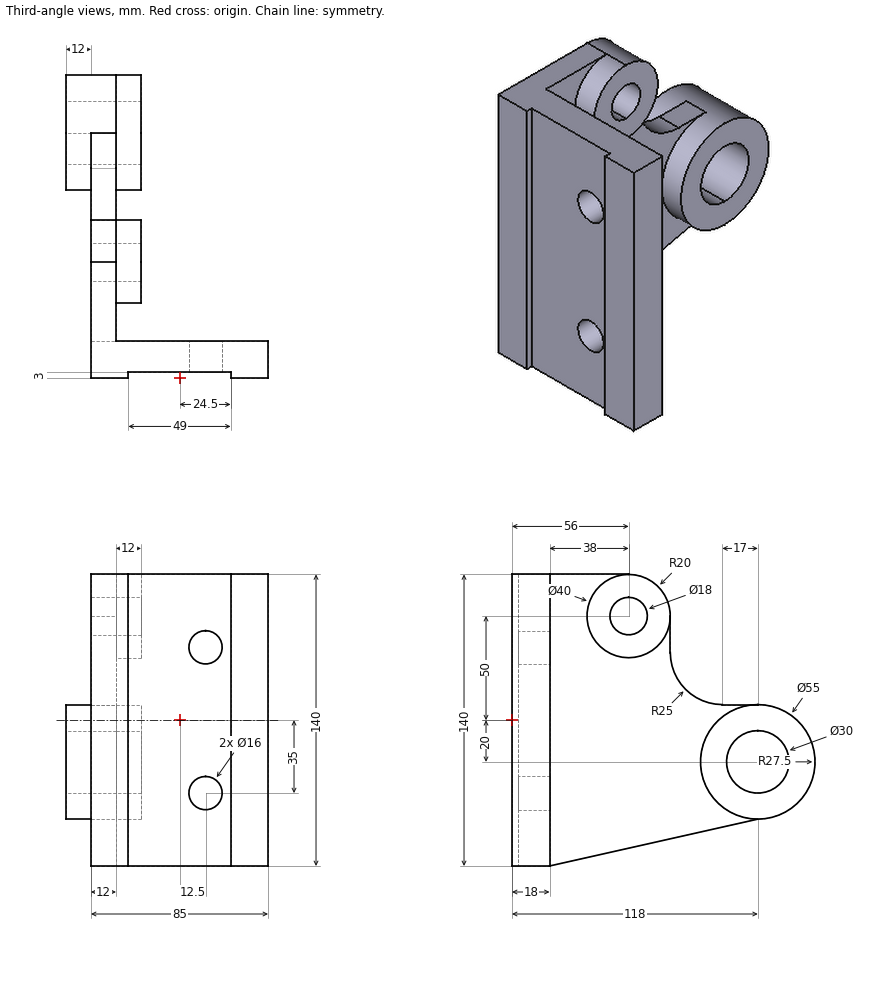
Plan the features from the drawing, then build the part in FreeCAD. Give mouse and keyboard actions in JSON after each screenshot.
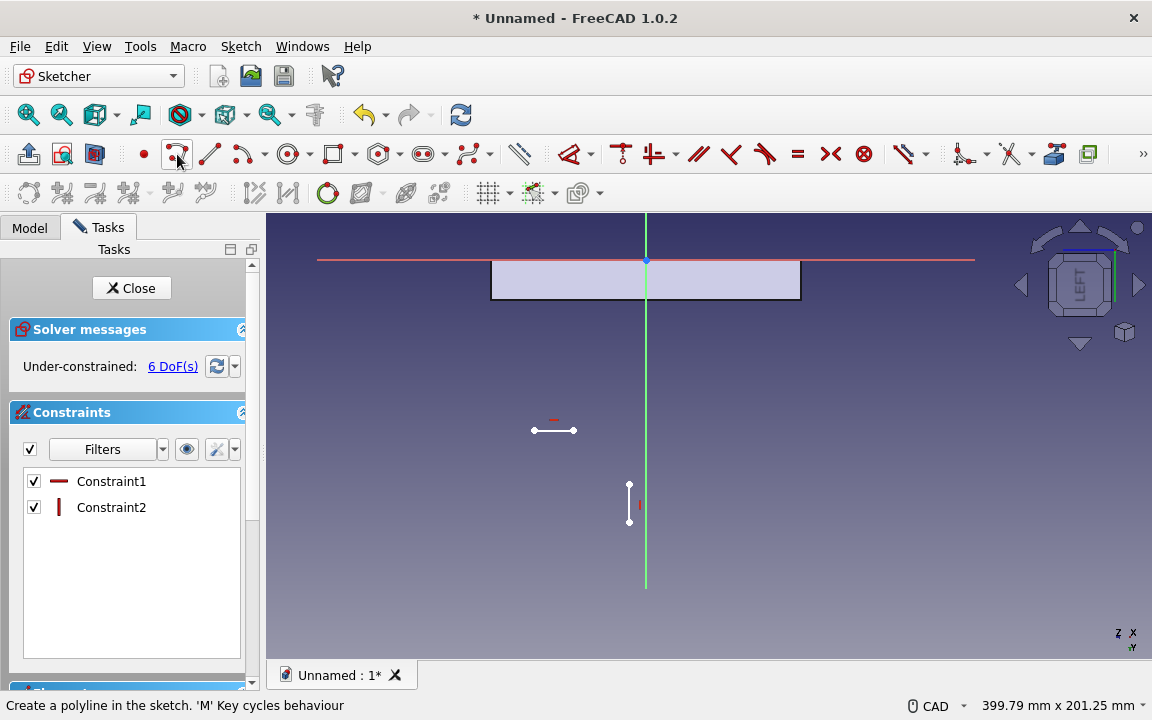
{"action": "left_click", "coordinate": [751, 522]}
{"action": "left_click", "coordinate": [801, 300]}
{"action": "left_click", "coordinate": [491, 300]}
{"action": "left_click", "coordinate": [491, 385]}
{"action": "right_click", "coordinate": [491, 385]}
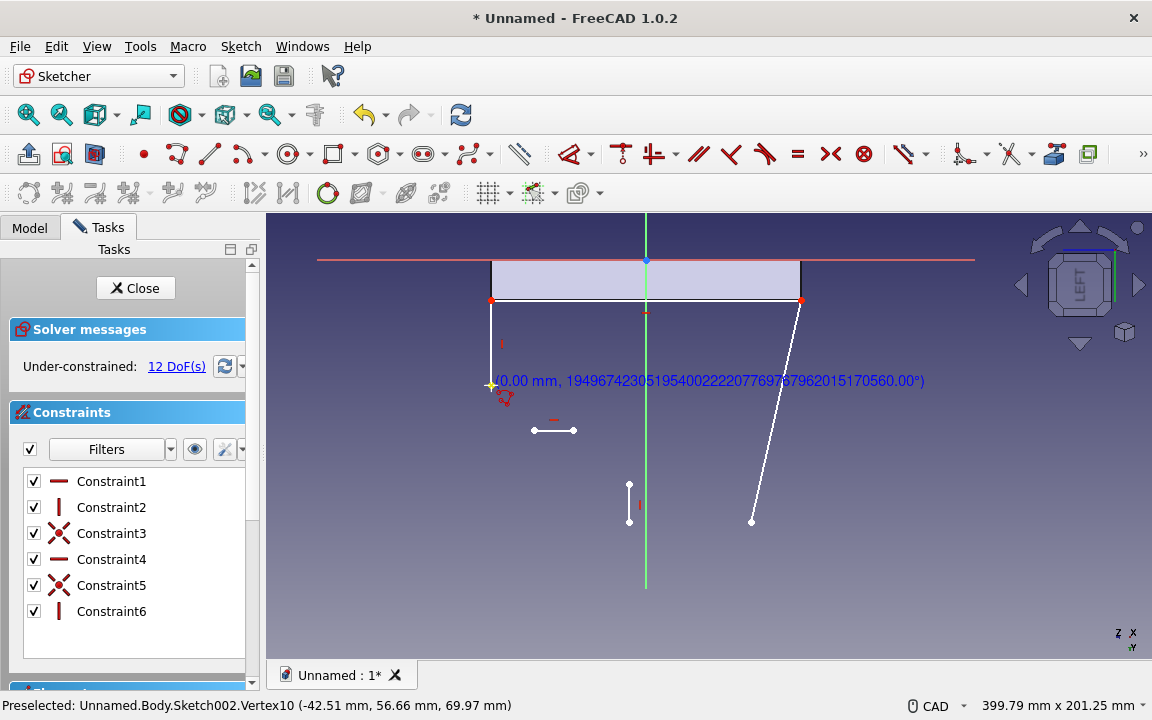
{"action": "key", "text": "g 3 a"}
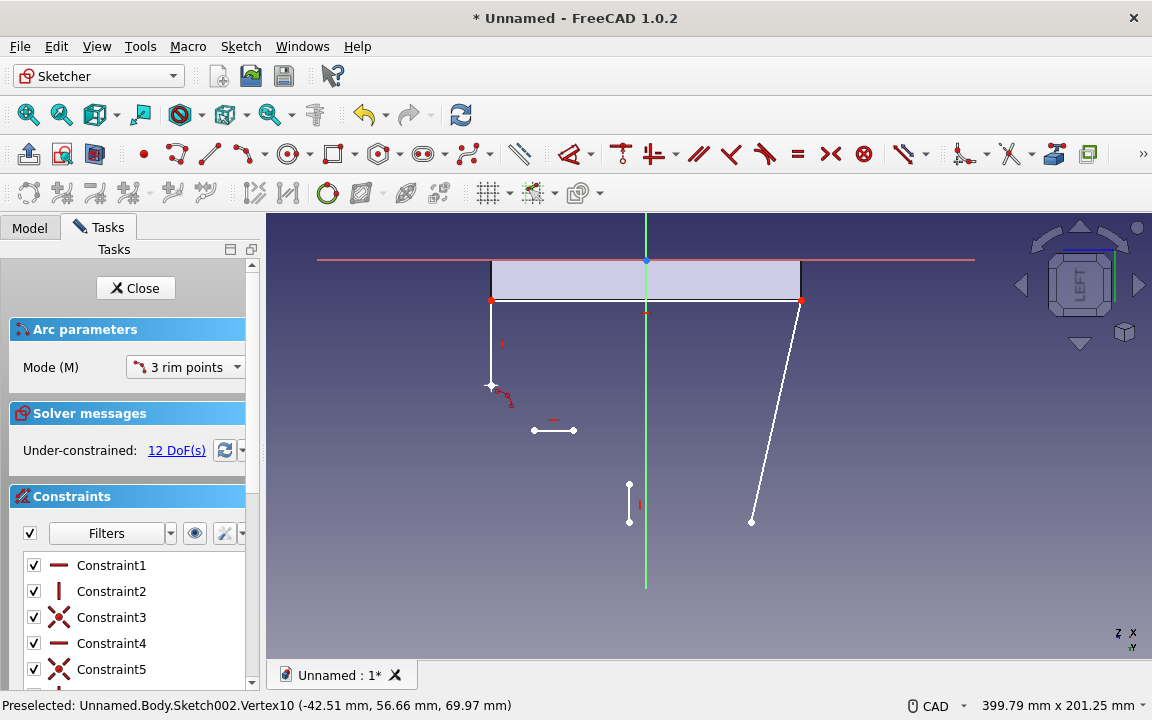
{"action": "left_click", "coordinate": [574, 431]}
{"action": "left_click", "coordinate": [629, 485]}
{"action": "left_click", "coordinate": [613, 445]}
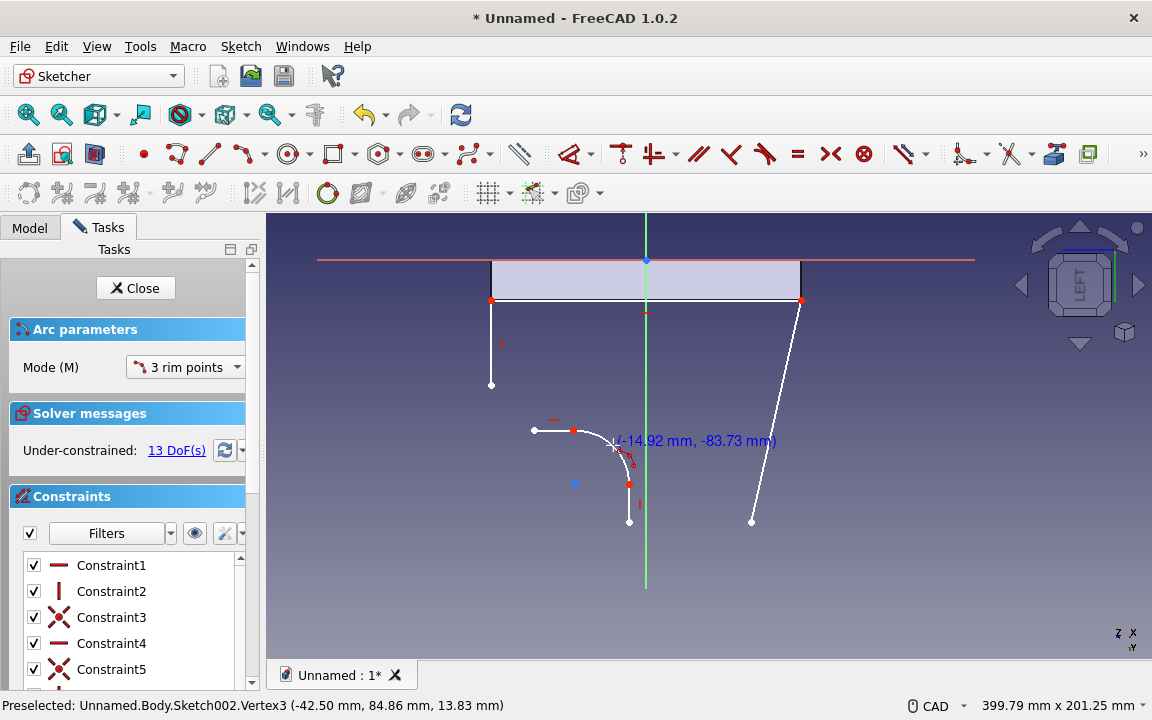
{"action": "left_click", "coordinate": [629, 523]}
{"action": "left_click", "coordinate": [751, 523]}
{"action": "left_click", "coordinate": [690, 583]}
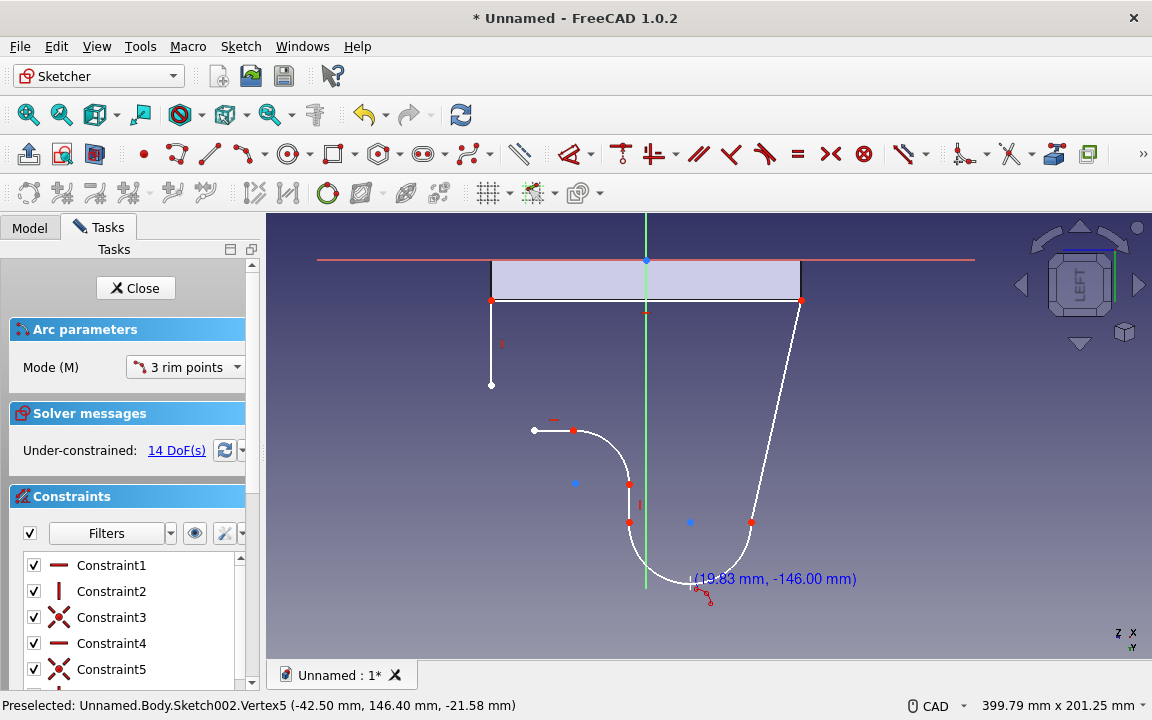
{"action": "left_click", "coordinate": [491, 386]}
{"action": "left_click", "coordinate": [535, 431]}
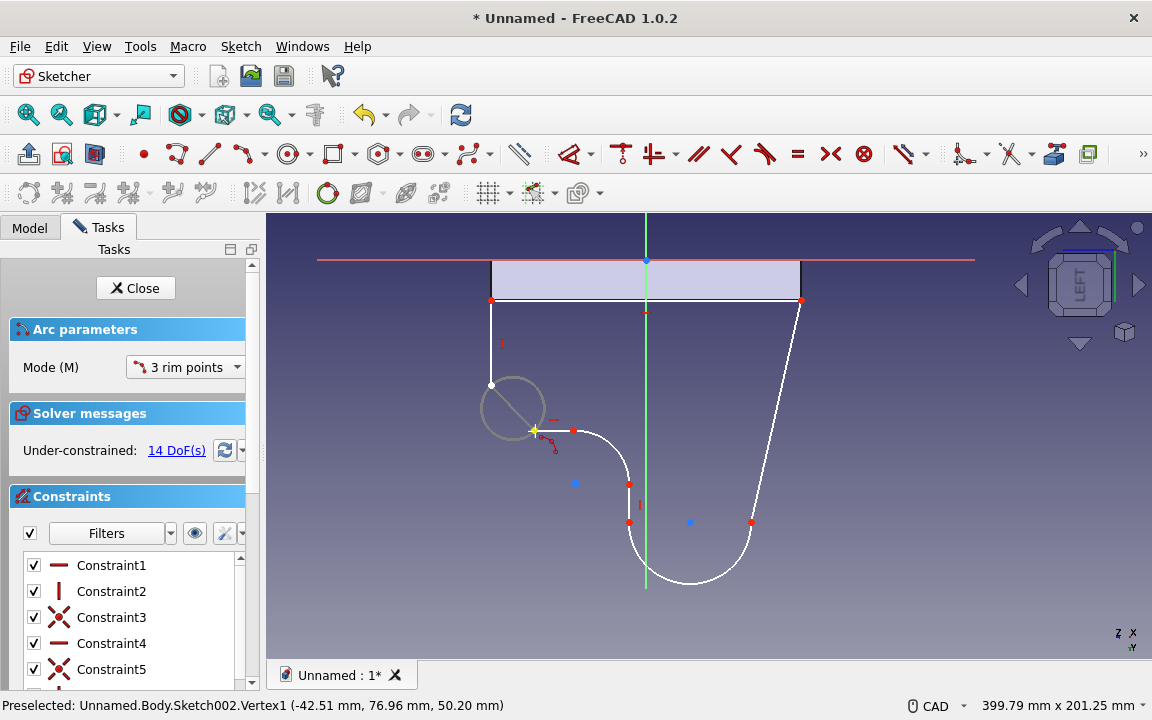
{"action": "scroll", "coordinate": [504, 416], "scroll_direction": "up", "scroll_amount": 2}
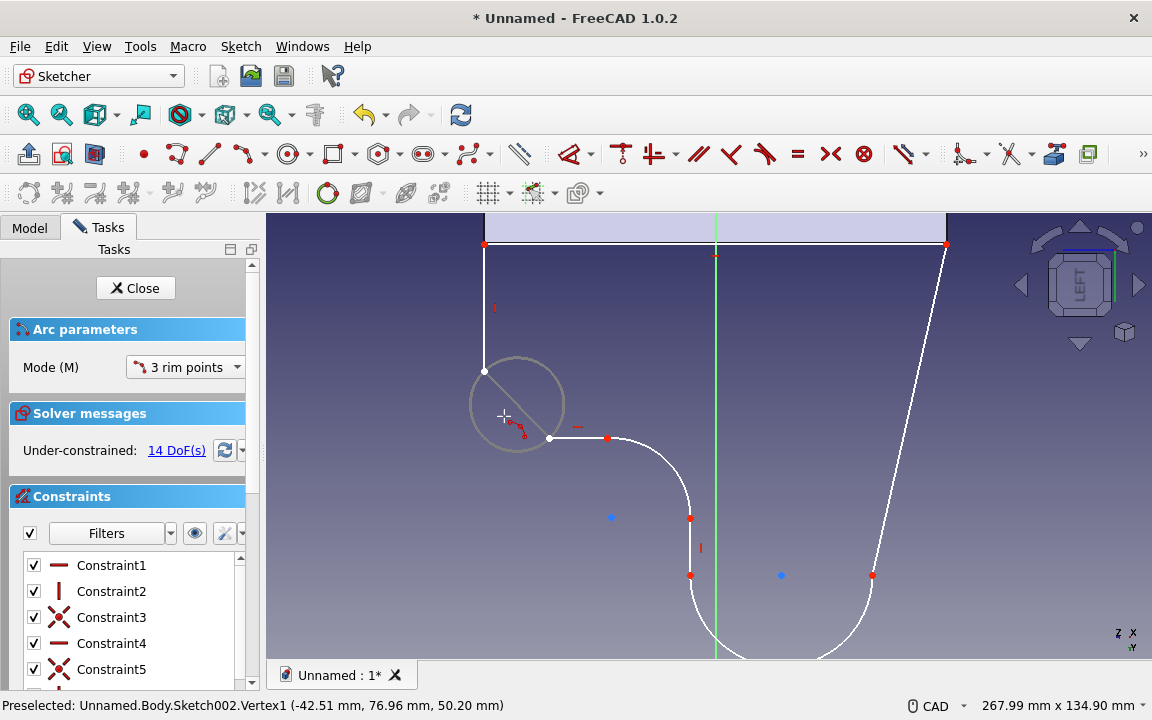
{"action": "left_click", "coordinate": [504, 416]}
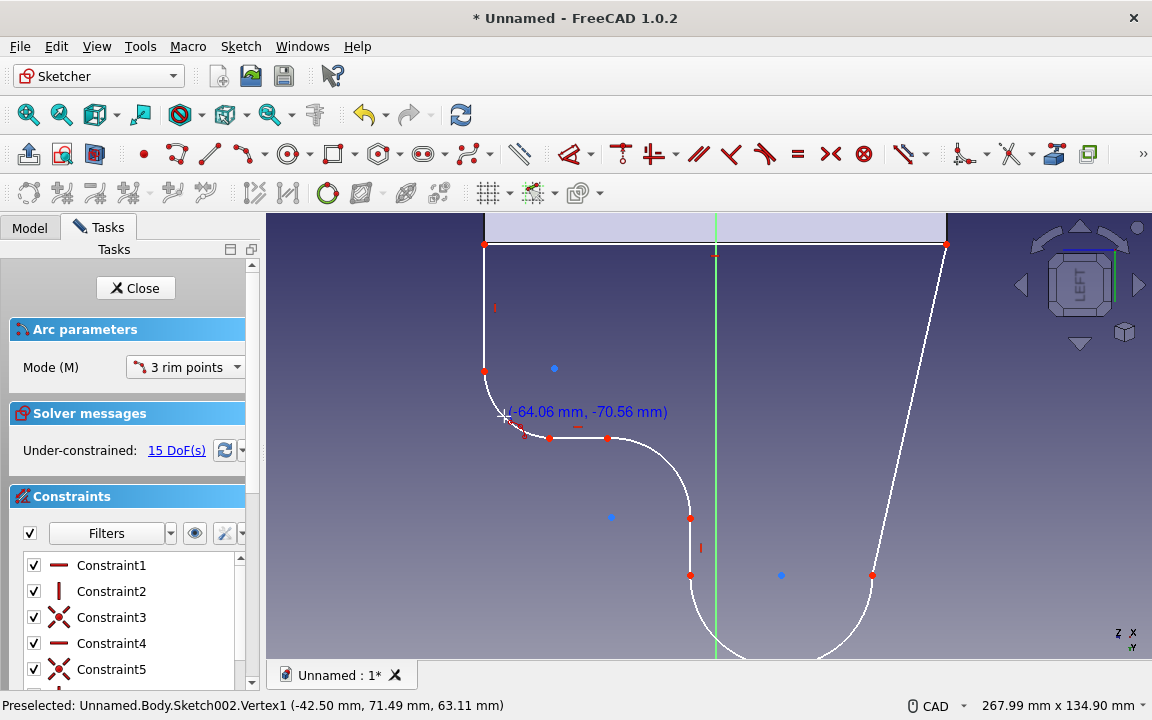
{"action": "key", "text": "g c"}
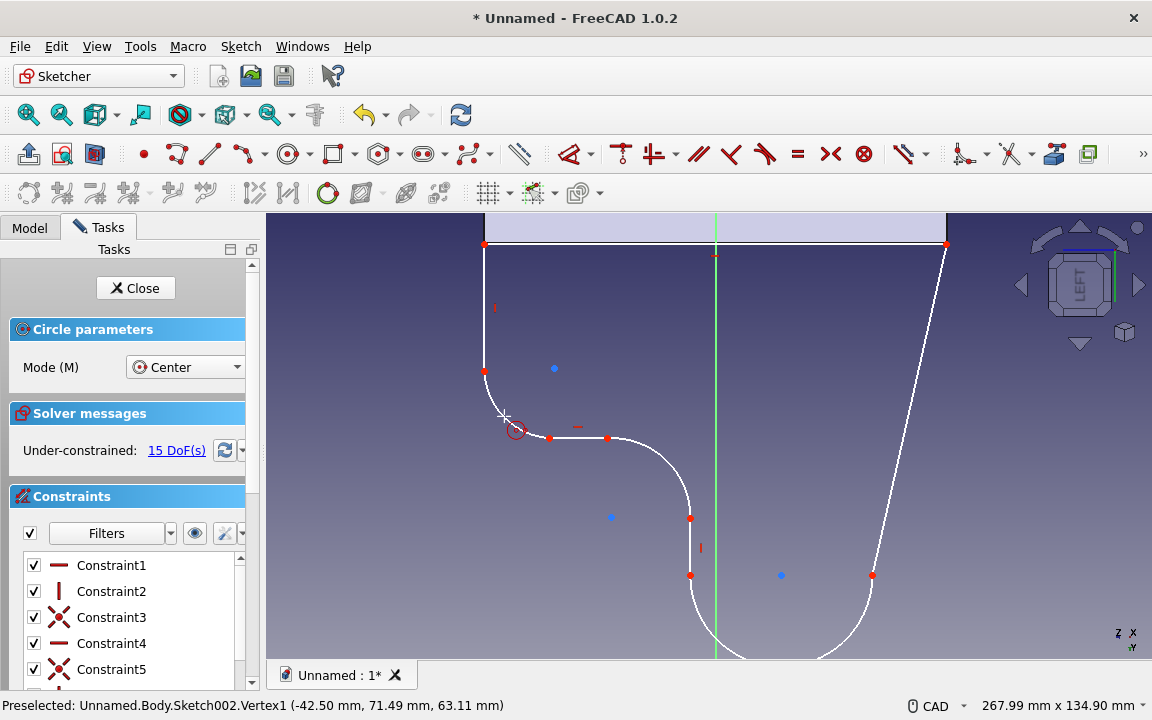
{"action": "left_click", "coordinate": [550, 369]}
{"action": "mouse_move", "coordinate": [572, 348]}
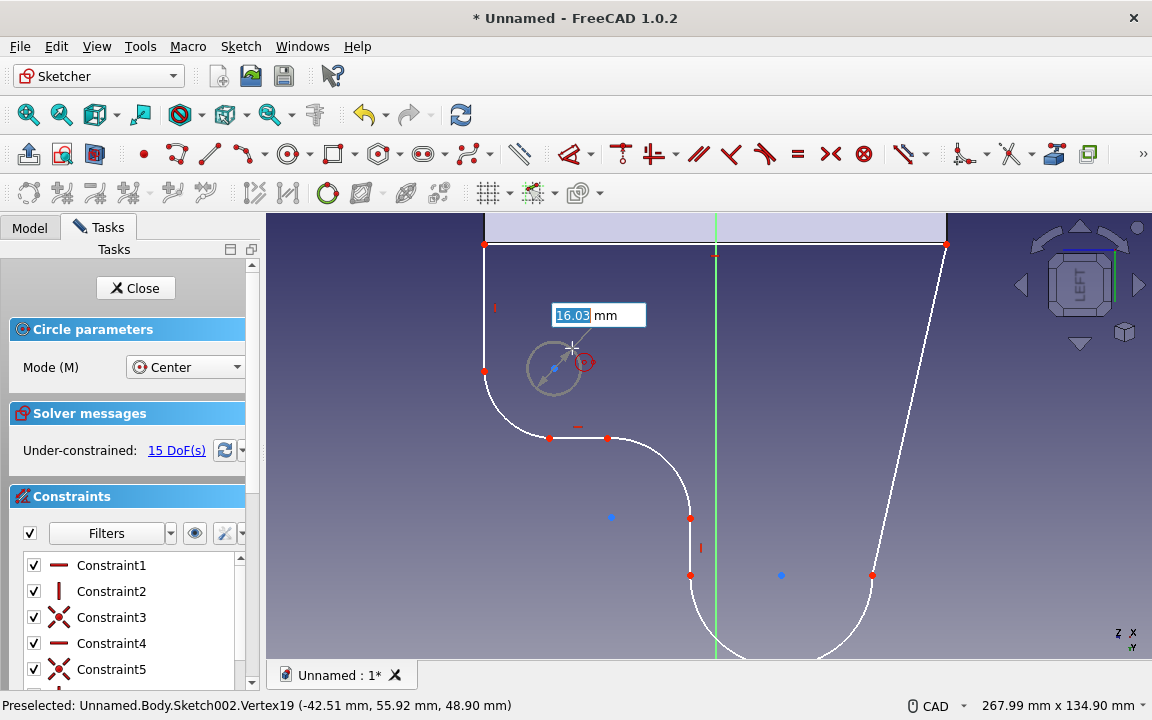
{"action": "type", "text": "18"}
{"action": "key", "text": "Return"}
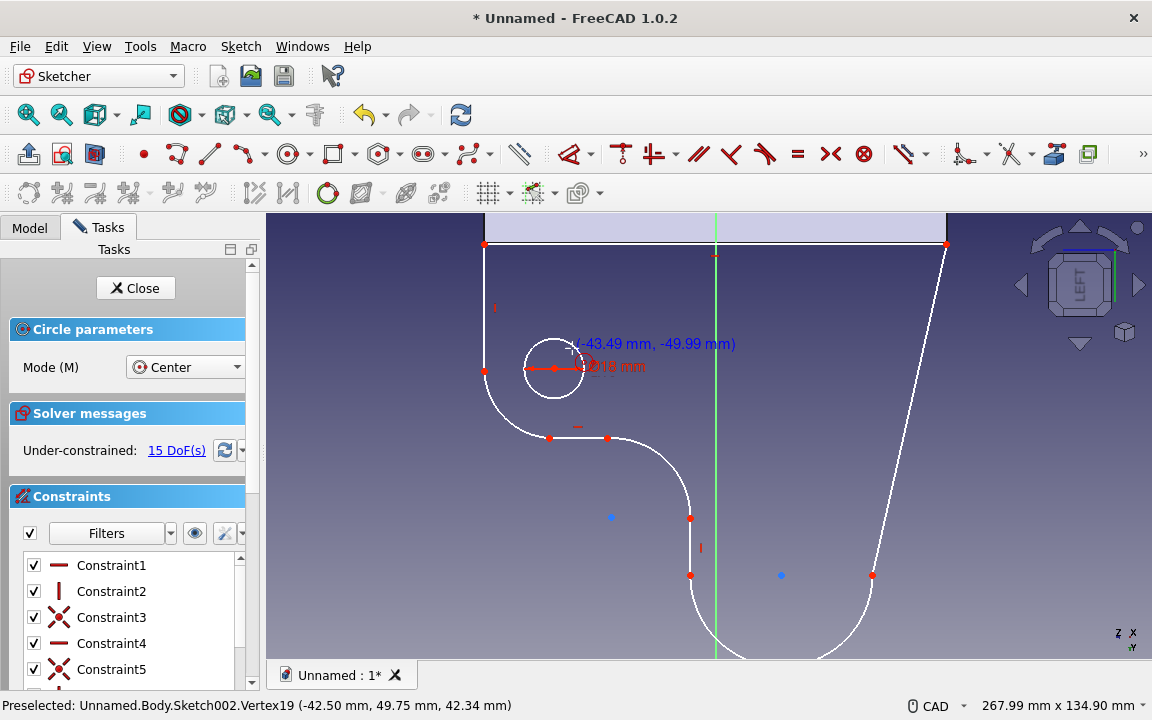
{"action": "left_click", "coordinate": [782, 574]}
{"action": "mouse_move", "coordinate": [817, 539]}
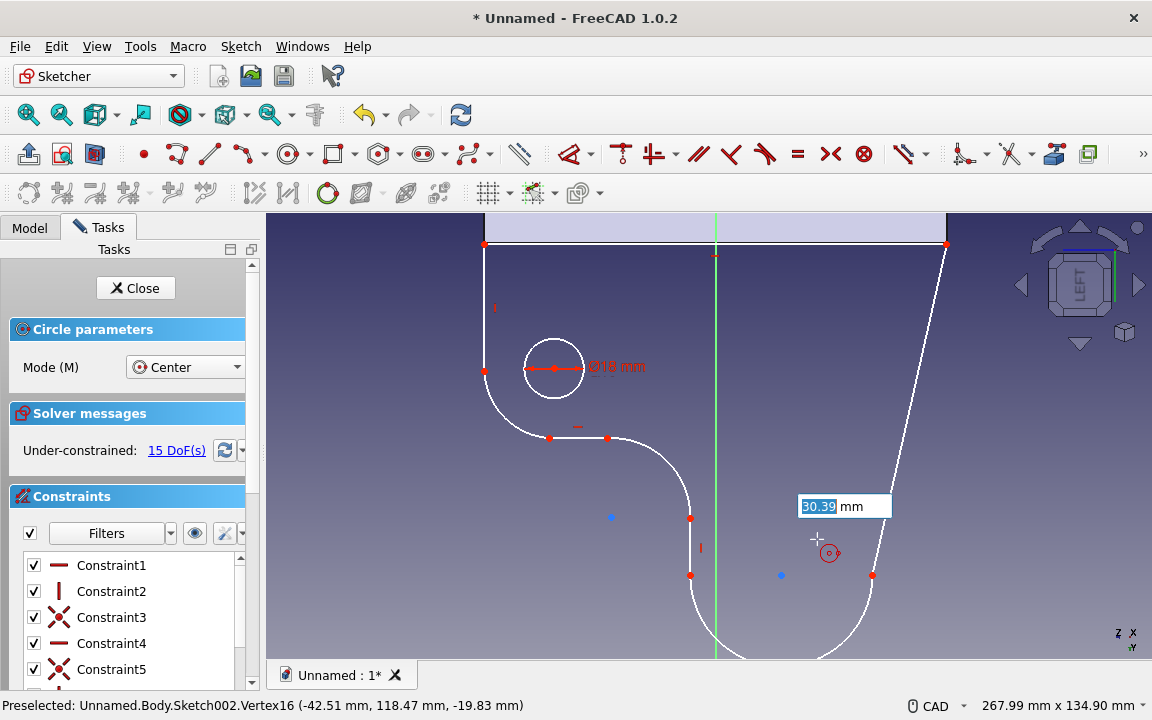
{"action": "type", "text": "30"}
{"action": "key", "text": "Return"}
{"action": "key", "text": "Escape"}